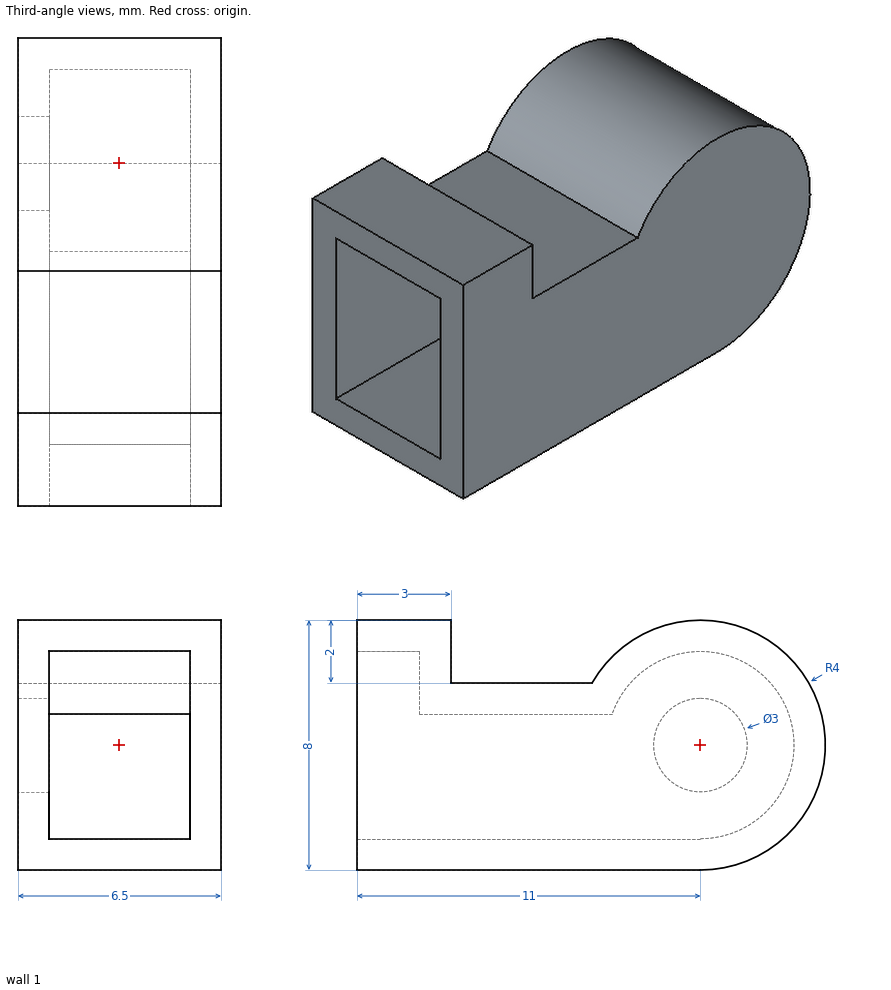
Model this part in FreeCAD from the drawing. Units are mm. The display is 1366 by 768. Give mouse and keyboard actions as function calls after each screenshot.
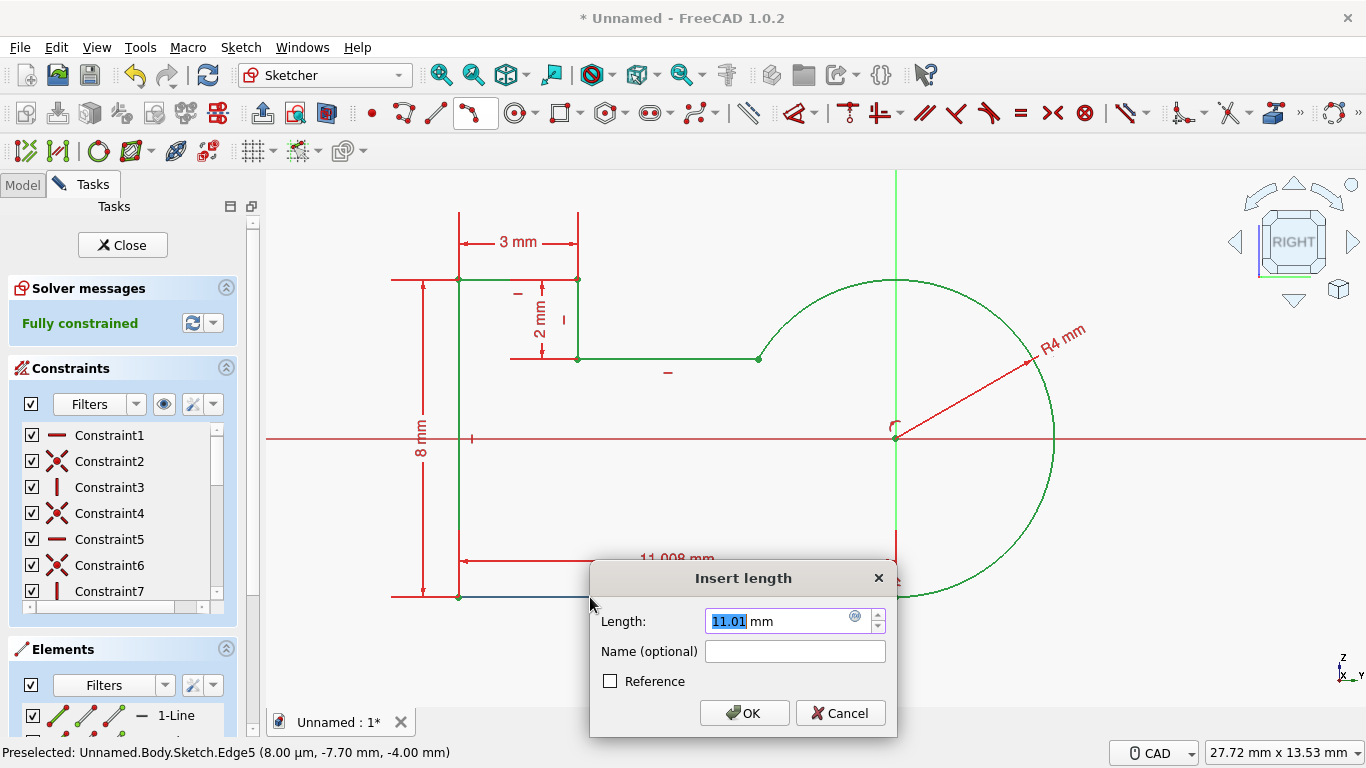
text(11)
key(Return)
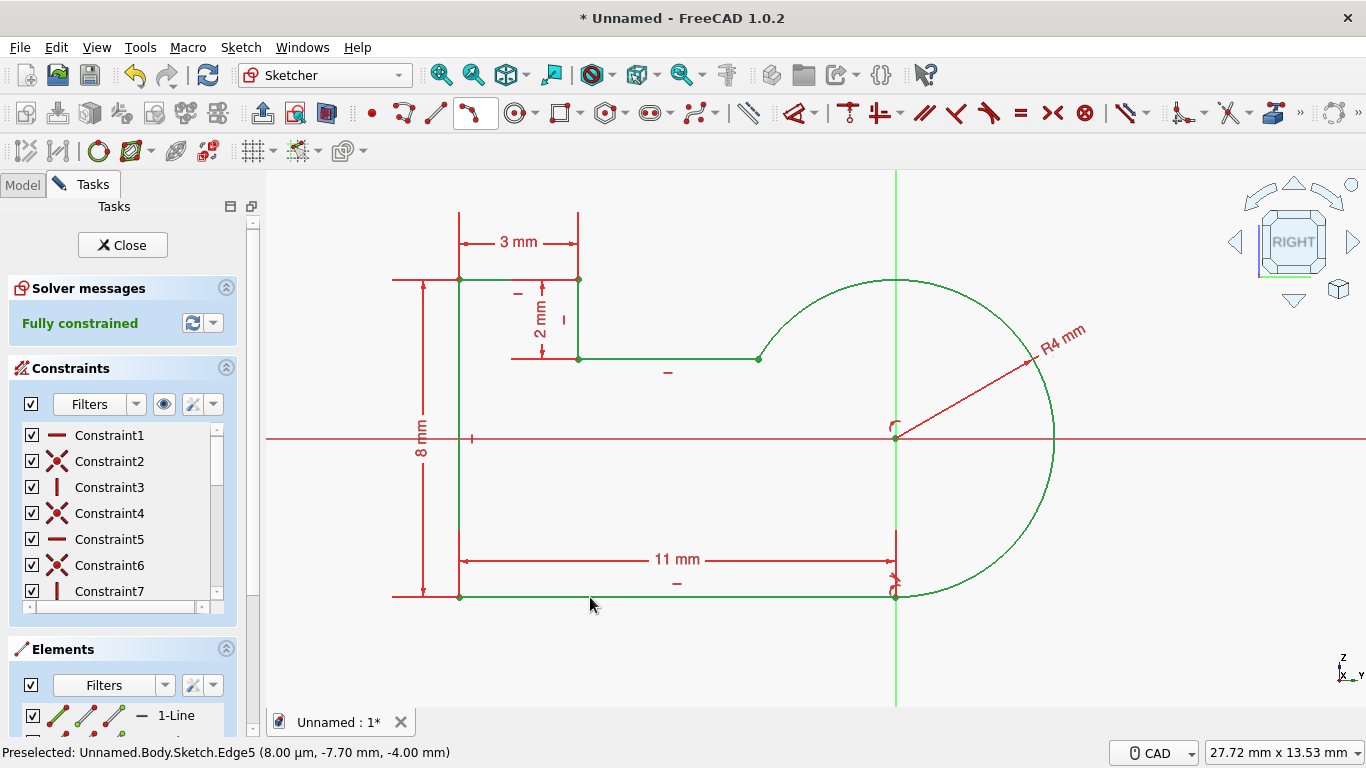
click(123, 245)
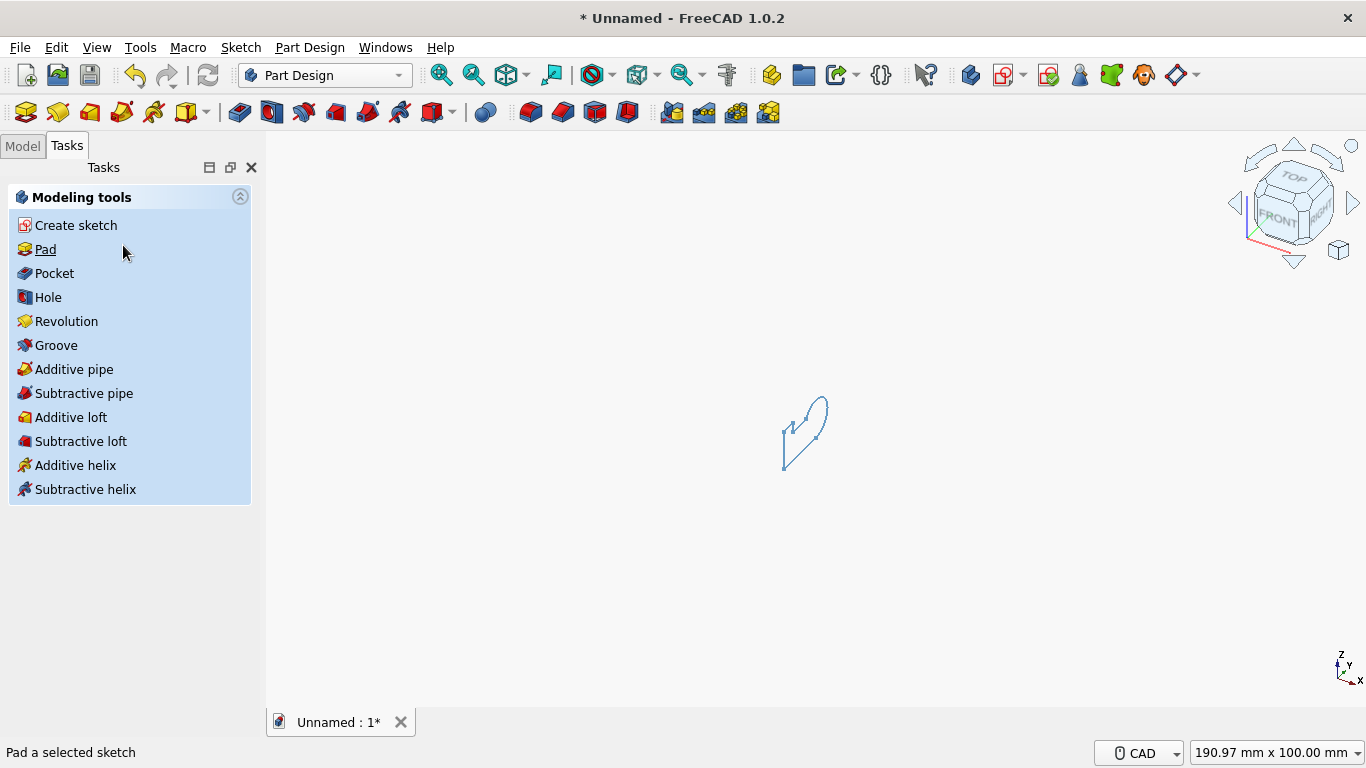
click(26, 112)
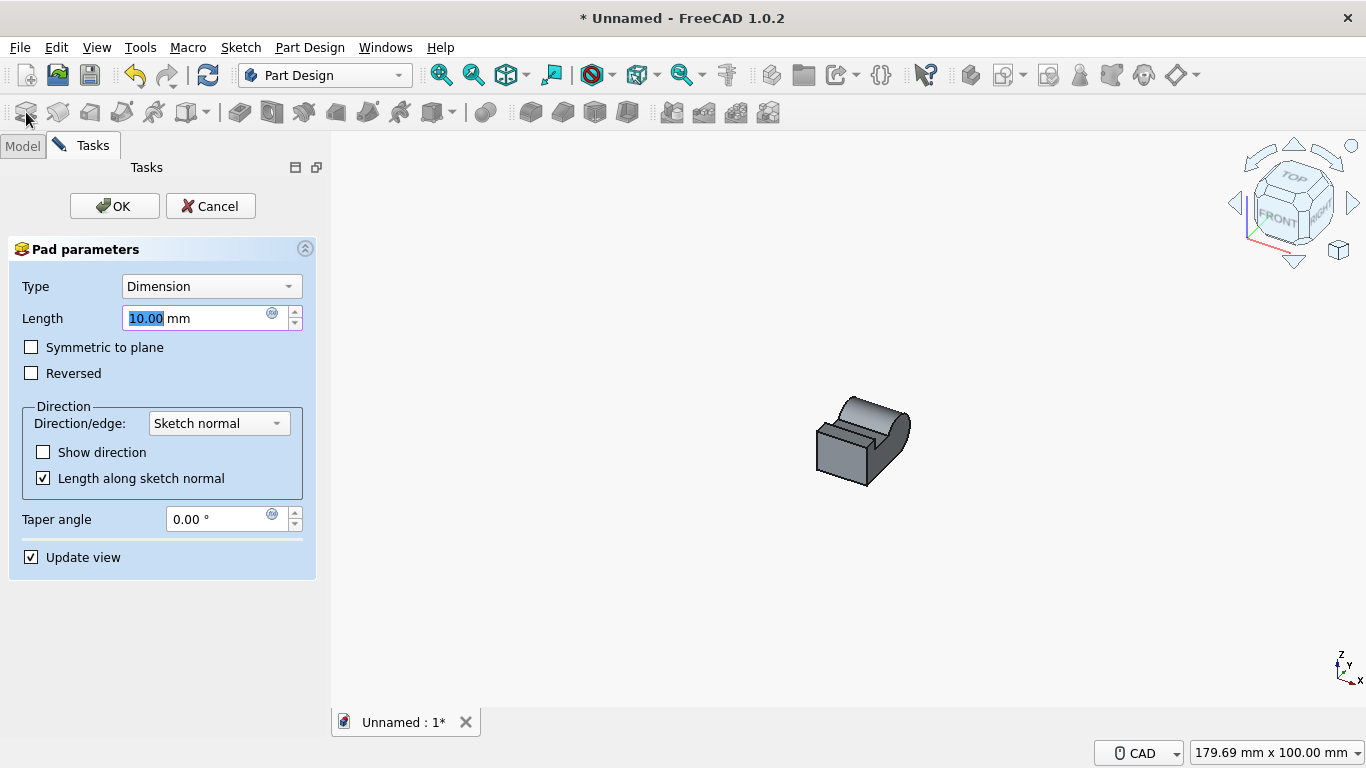
text(6.5)
key(Tab)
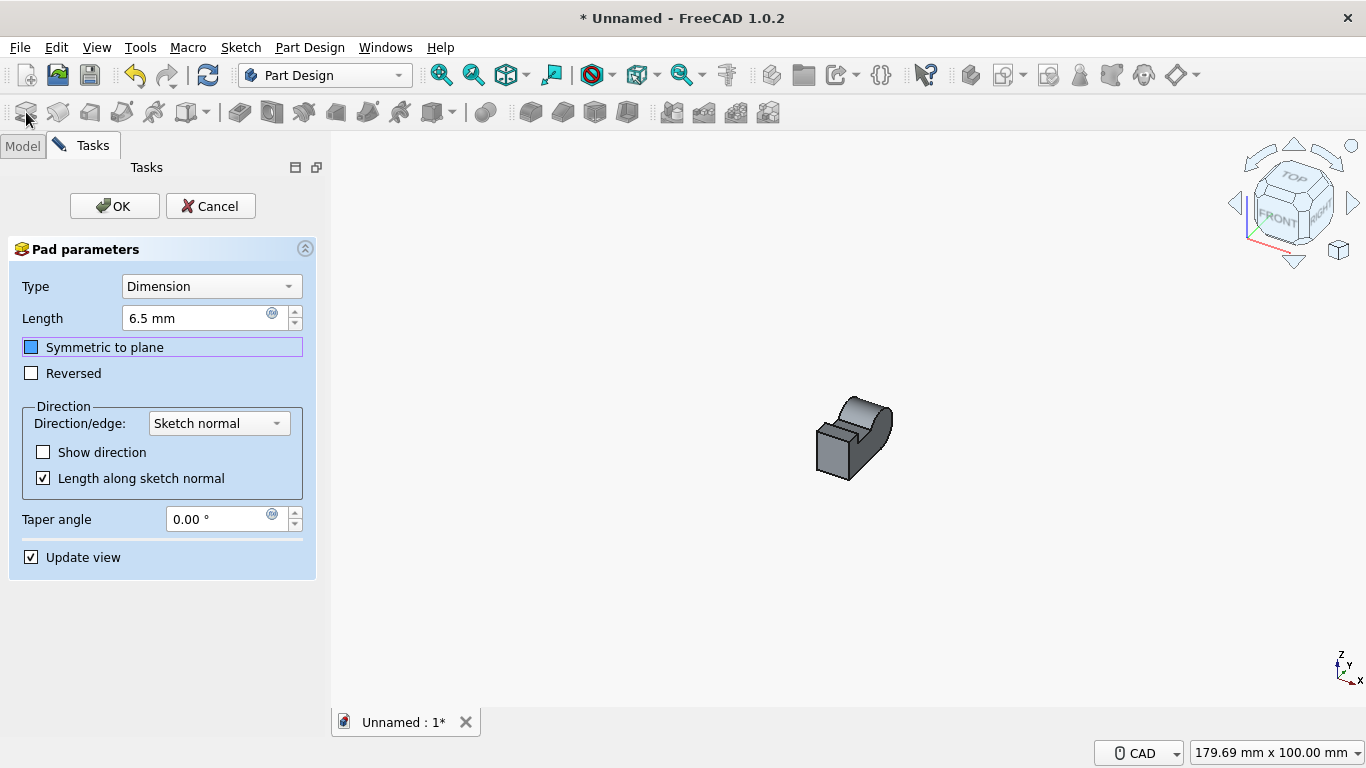
click(30, 347)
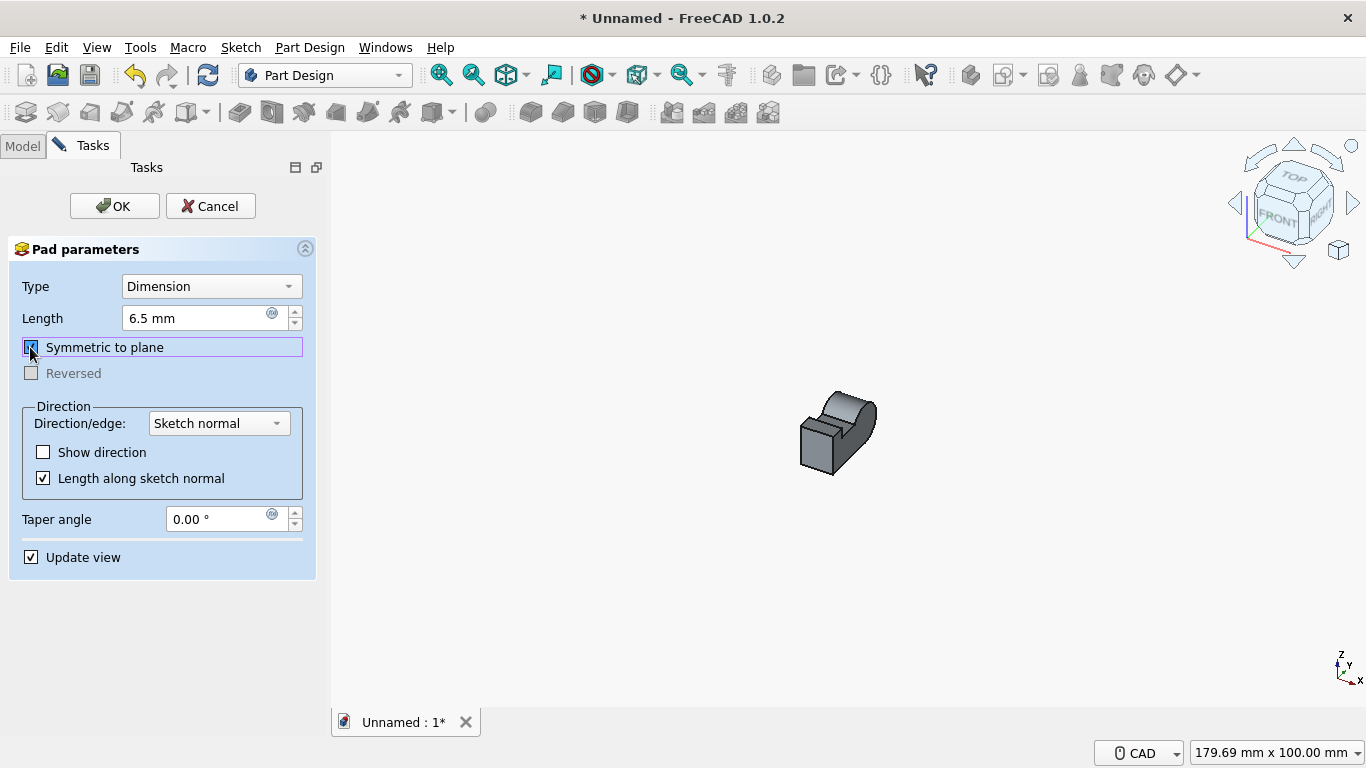
click(115, 206)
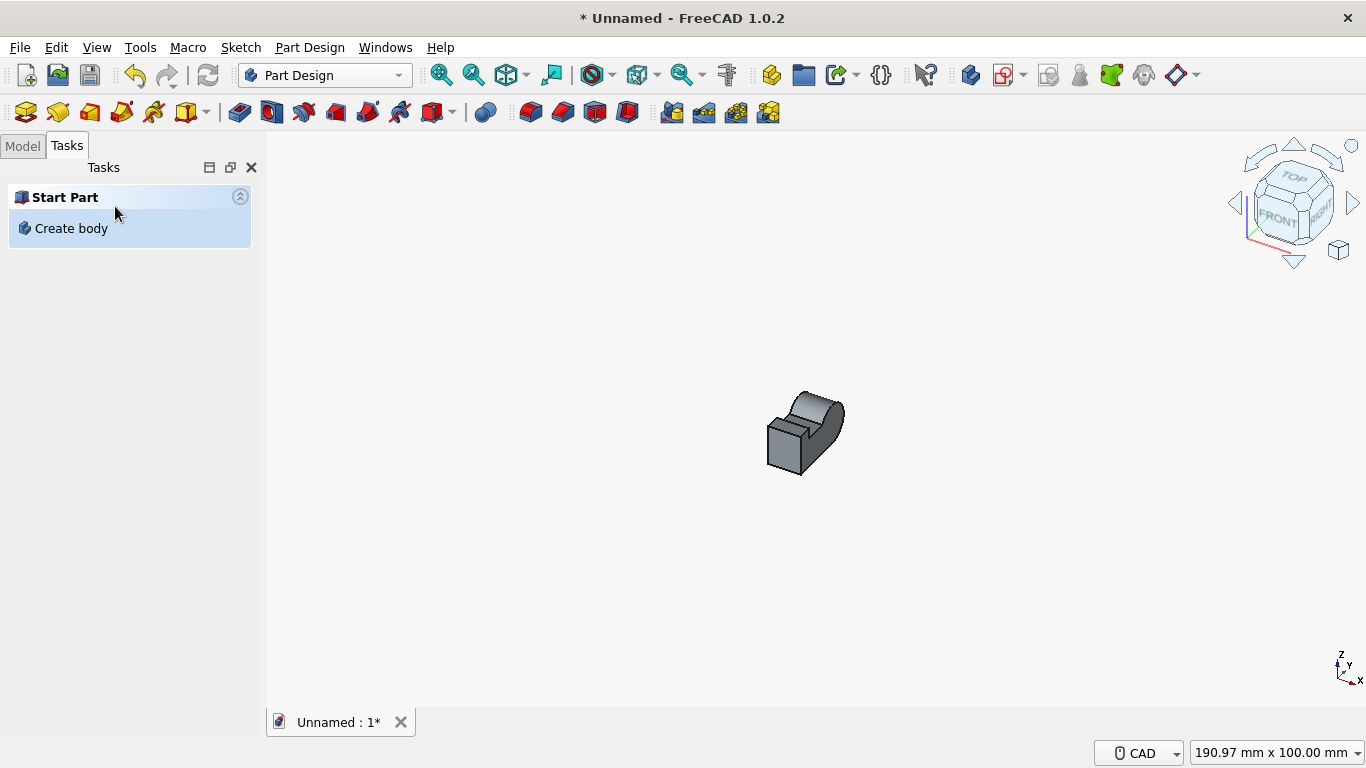
click(442, 76)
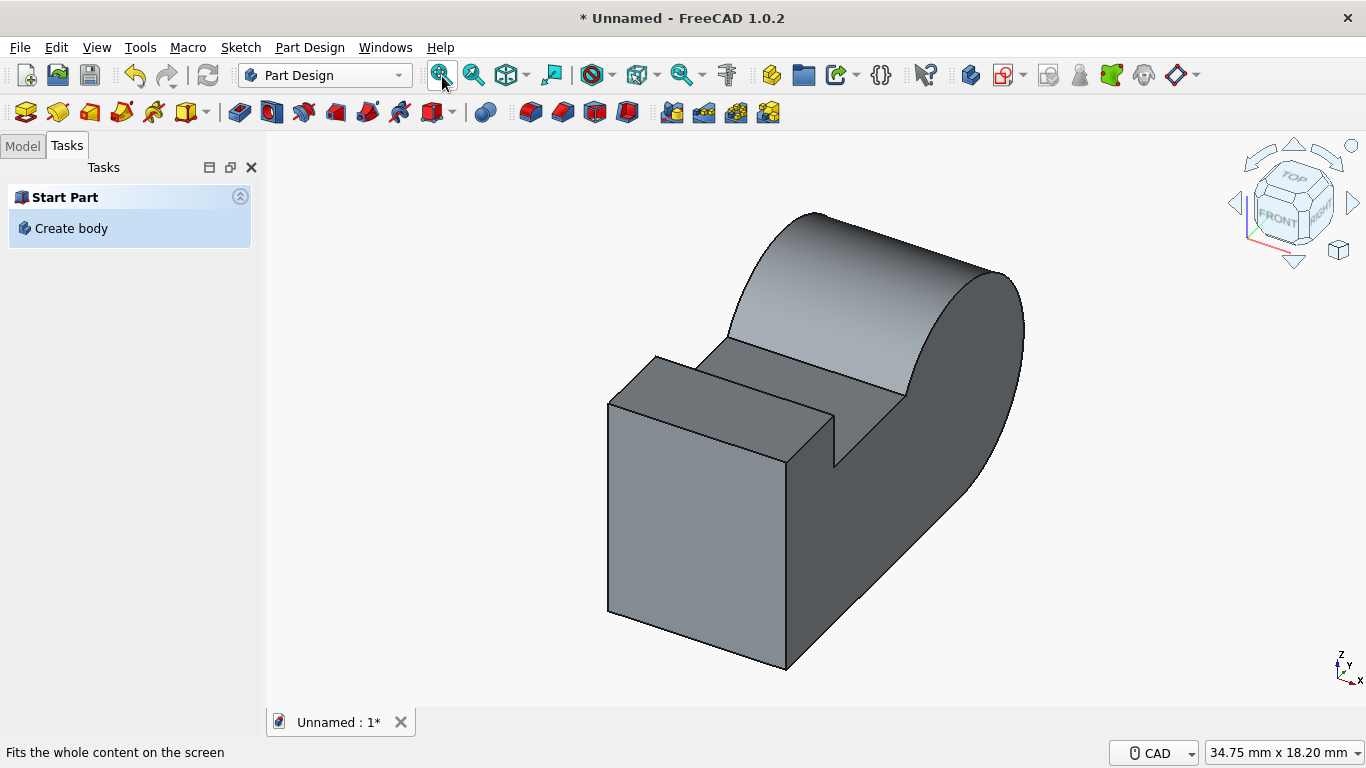
click(697, 536)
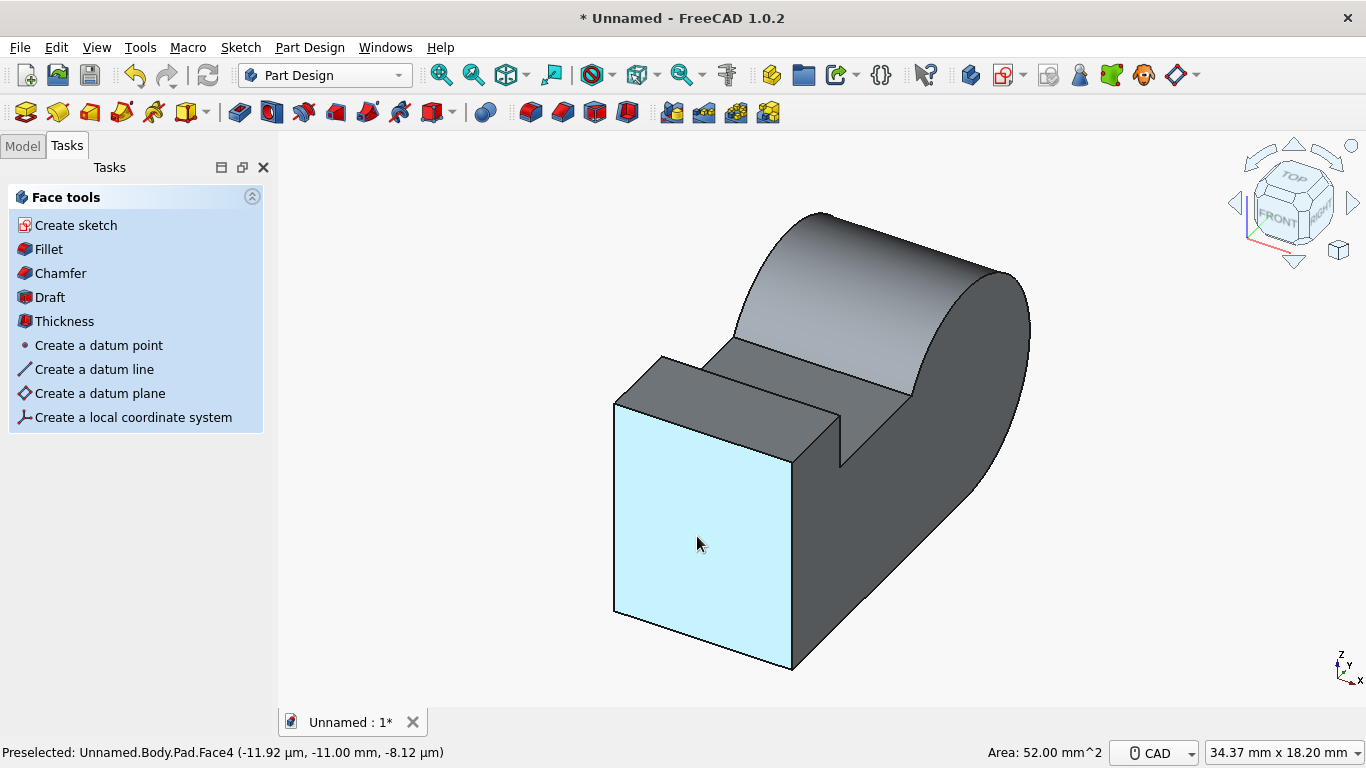
click(628, 112)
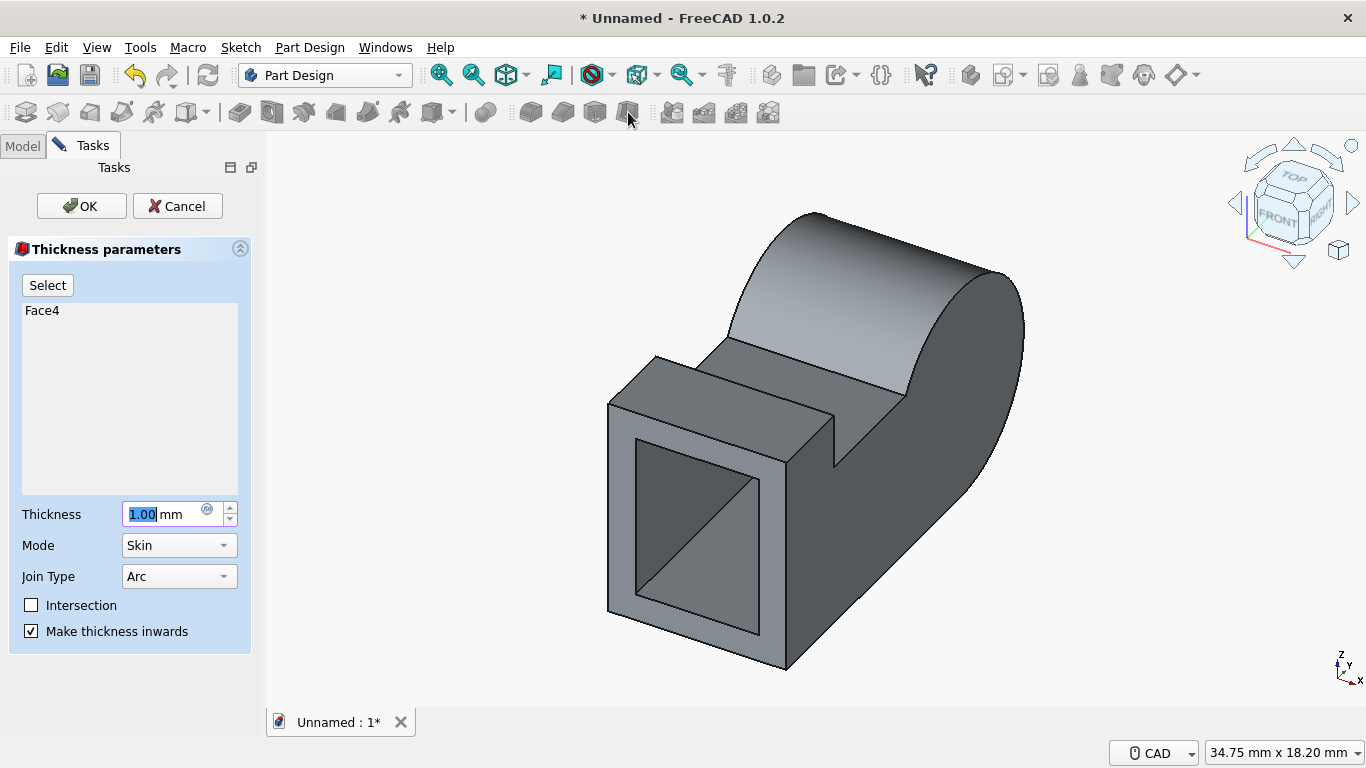
text(1)
key(Tab)